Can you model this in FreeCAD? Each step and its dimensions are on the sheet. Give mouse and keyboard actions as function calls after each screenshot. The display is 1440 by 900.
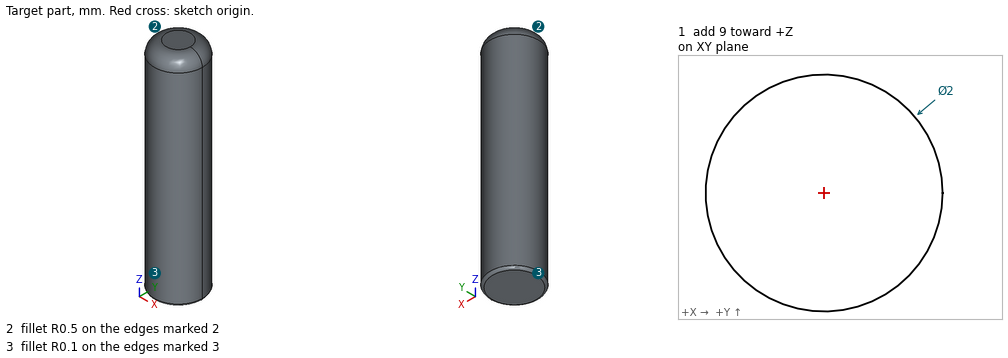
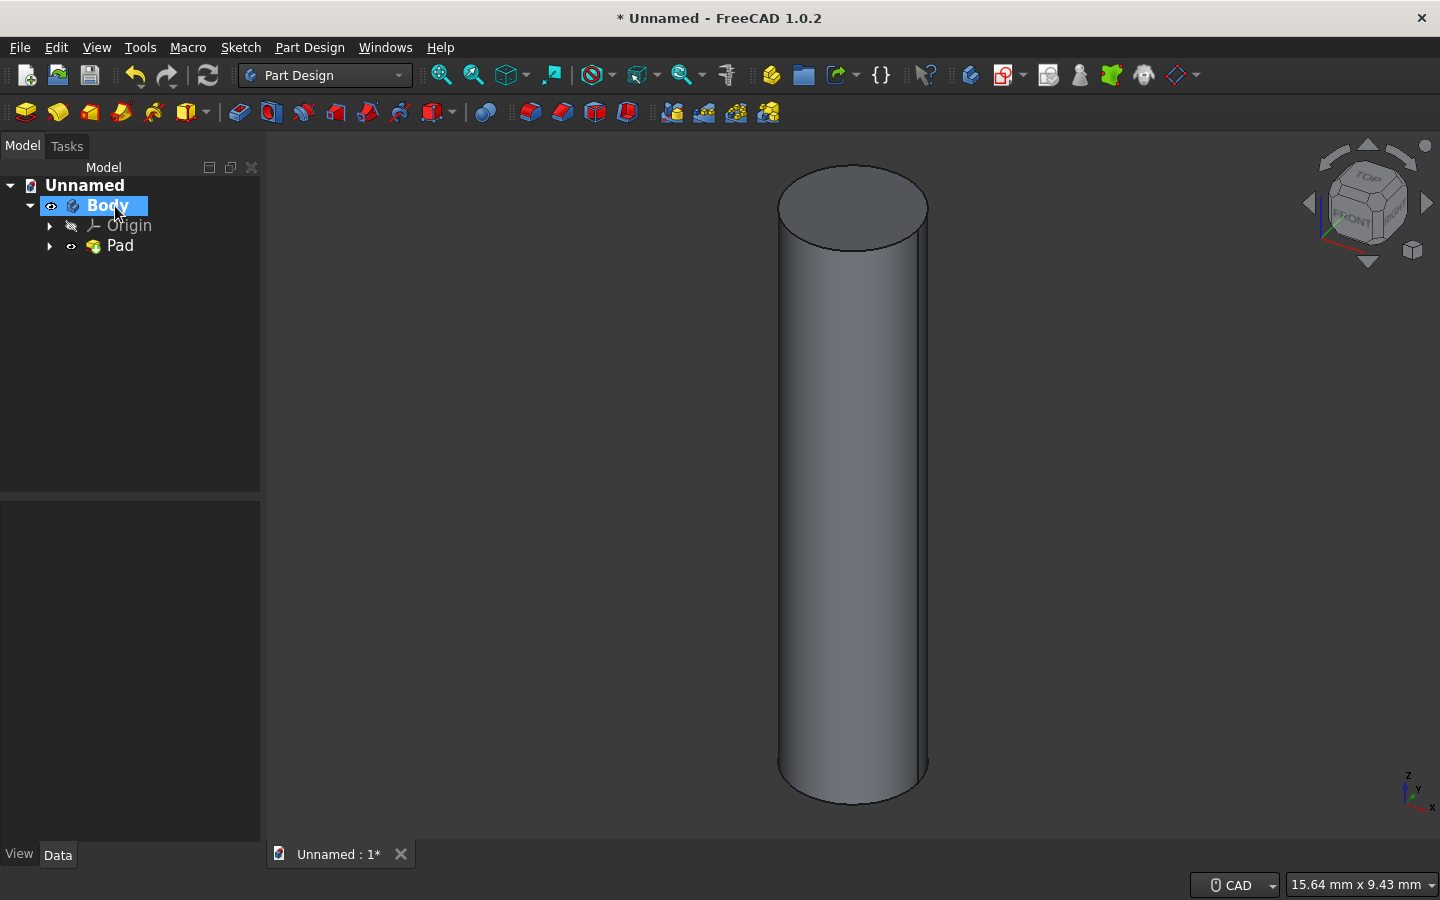
click(778, 212)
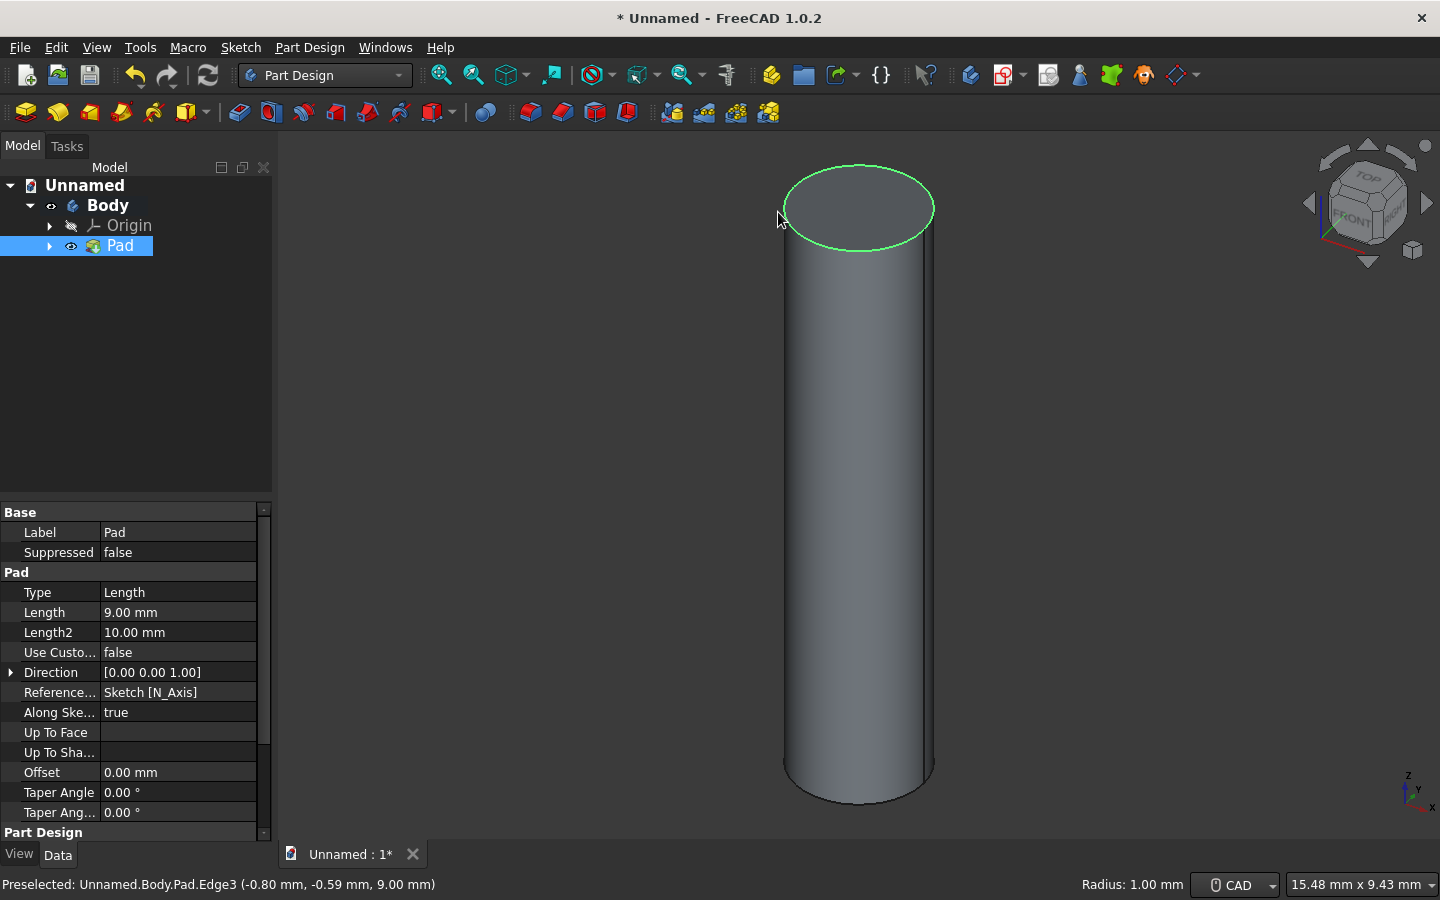
click(532, 112)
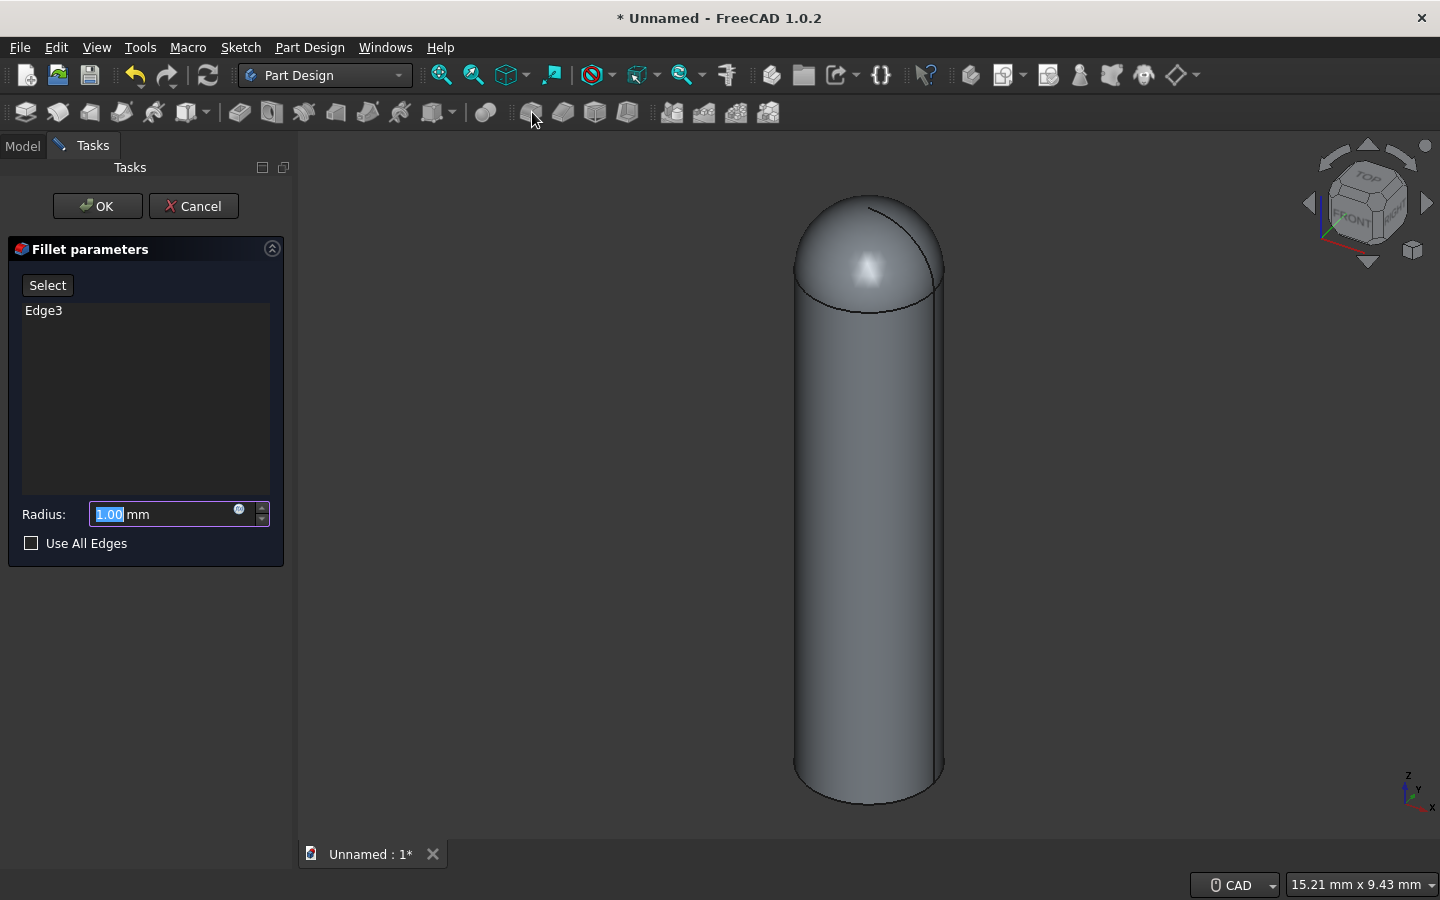
text(0.5)
key(Tab)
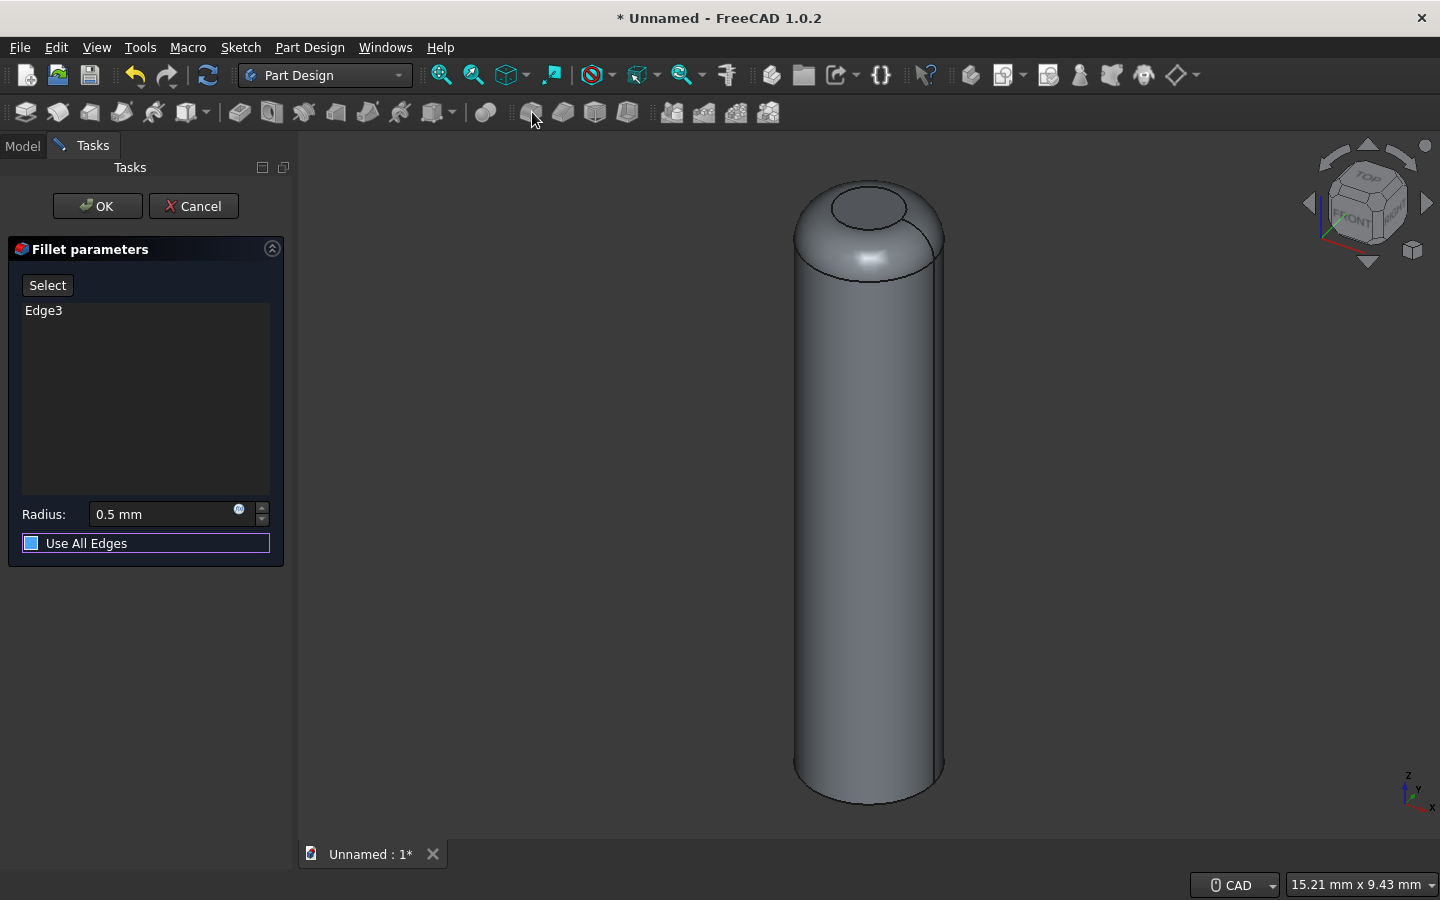
click(98, 206)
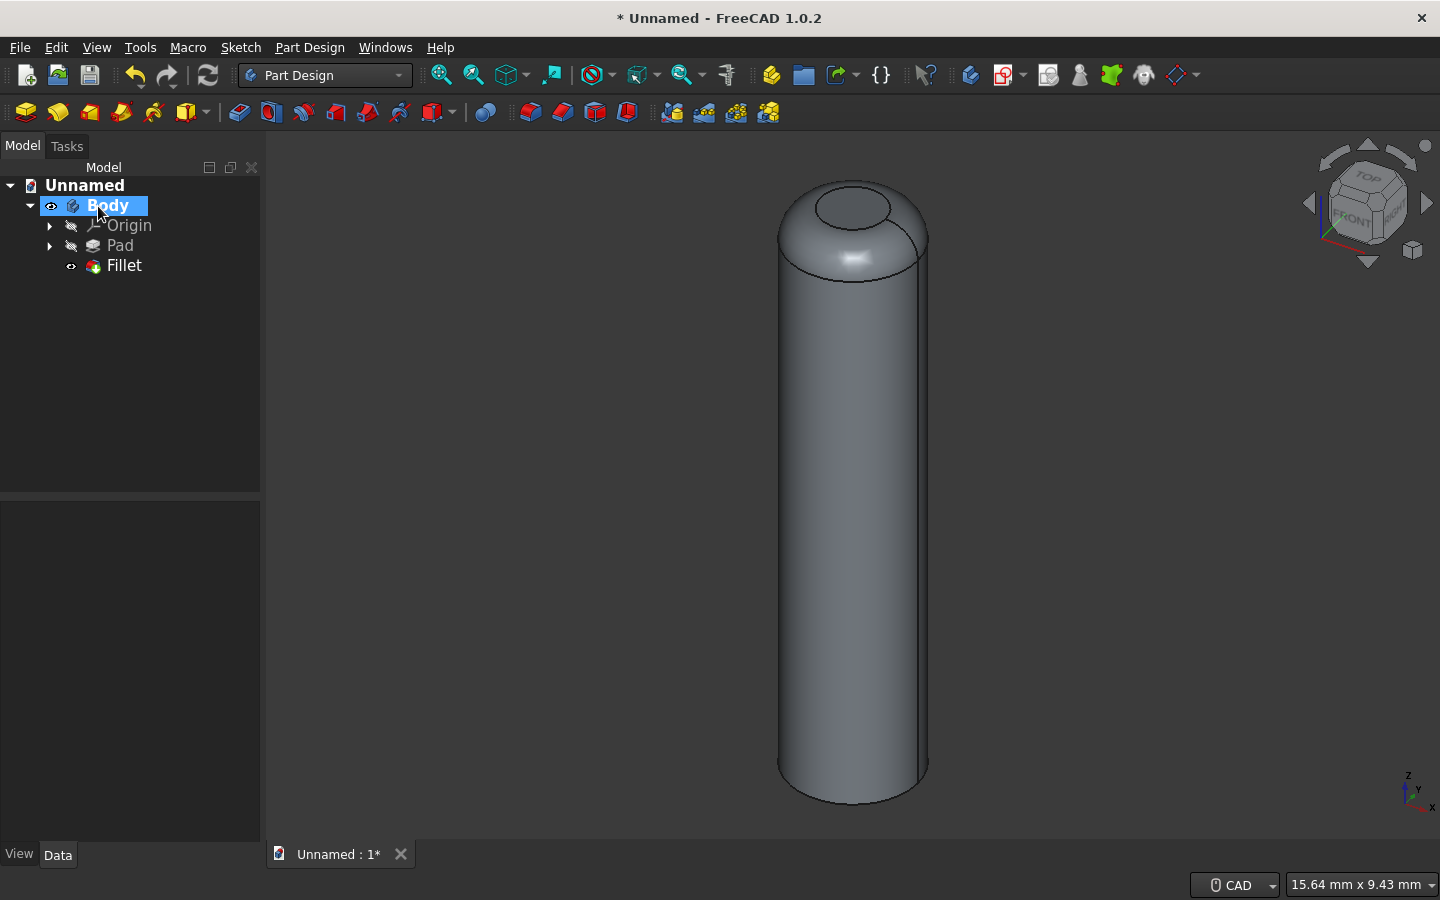
click(797, 790)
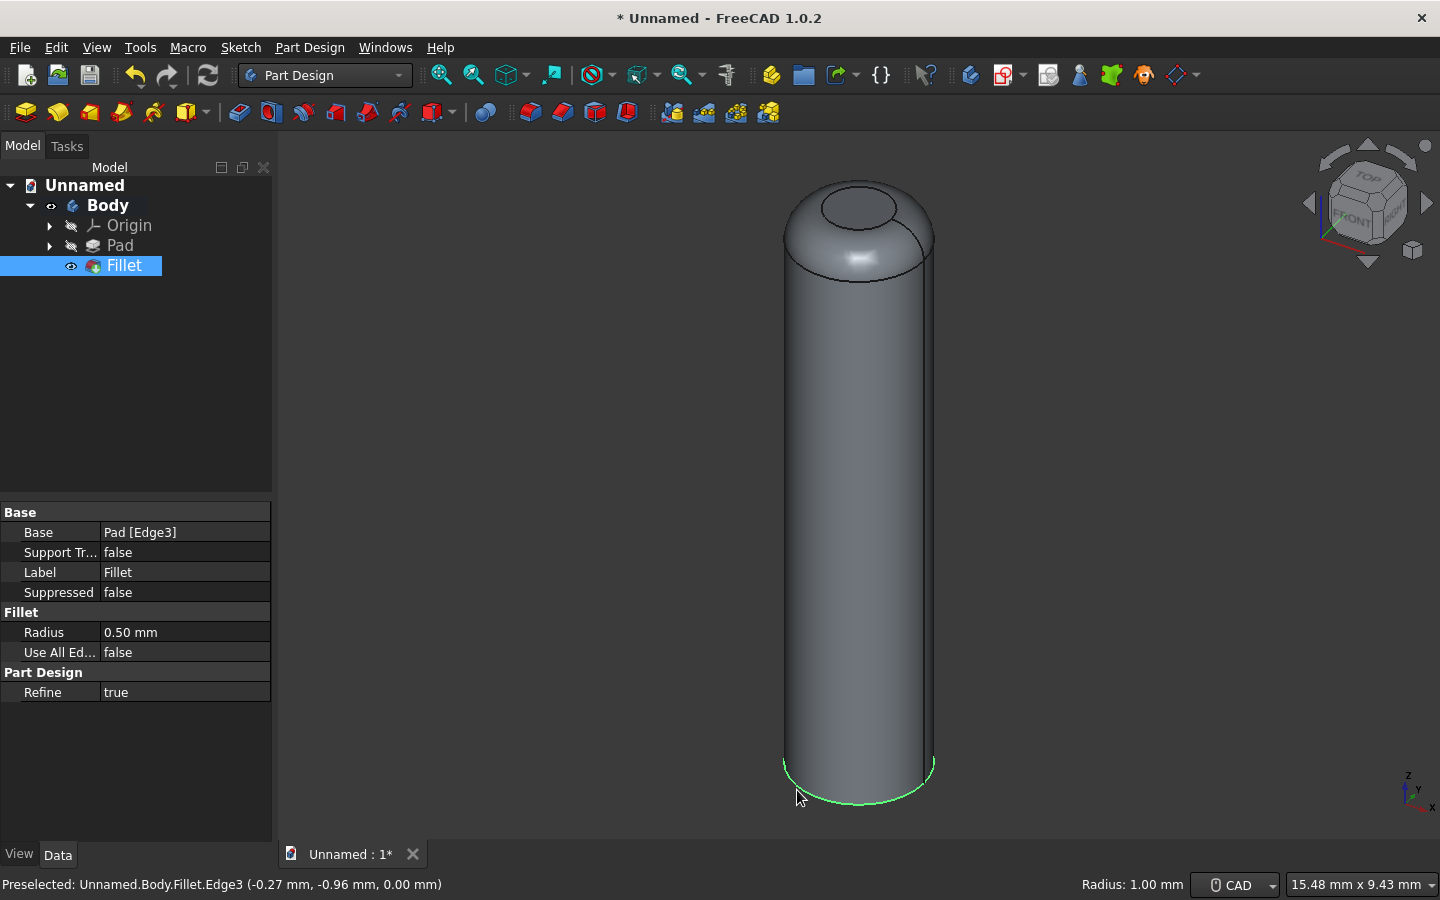
click(532, 112)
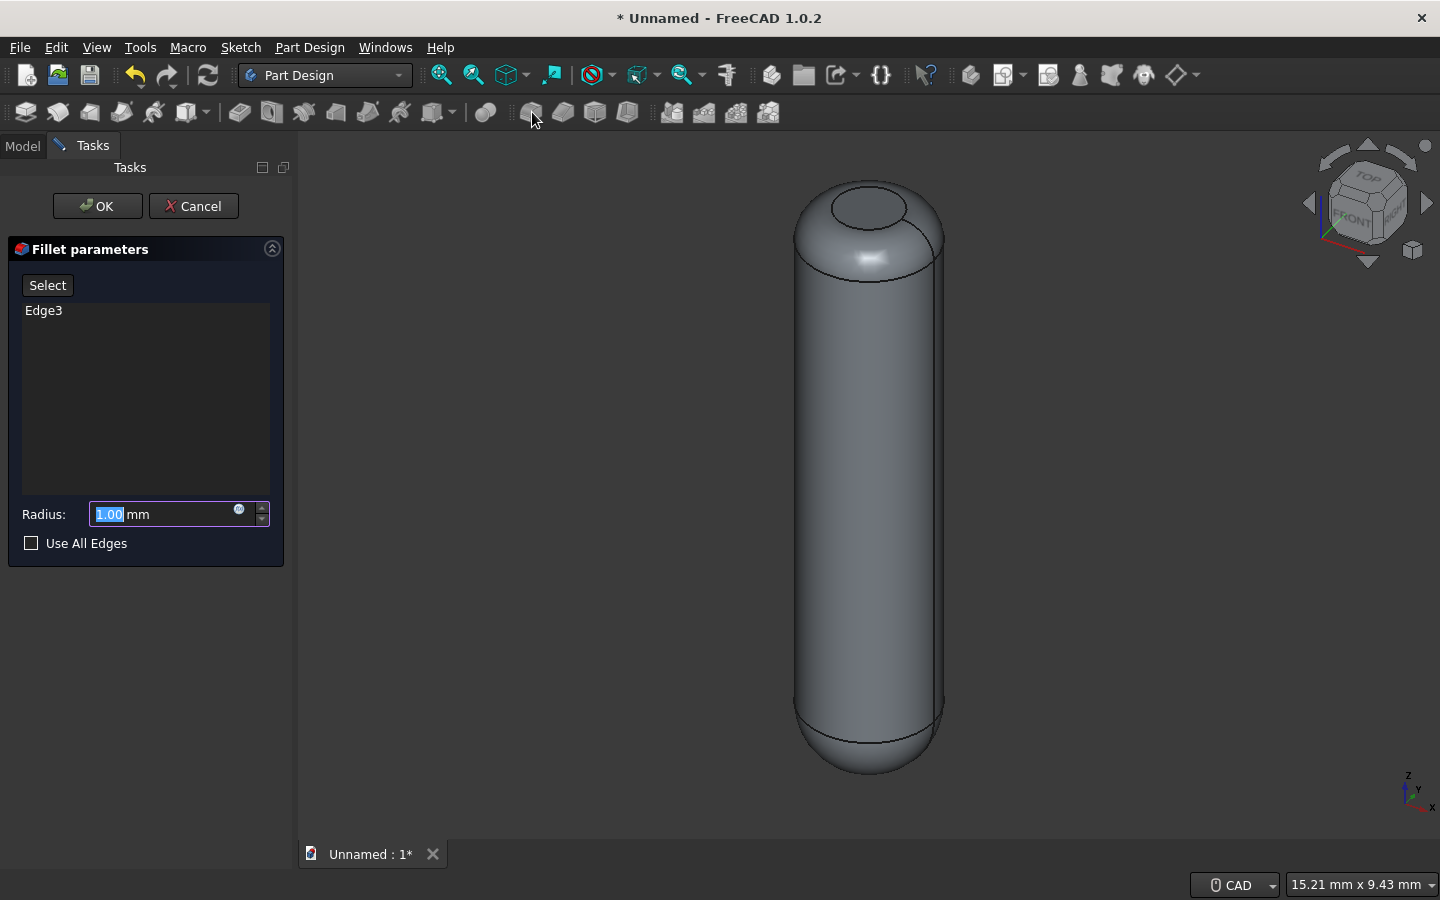
text(0.1)
key(Tab)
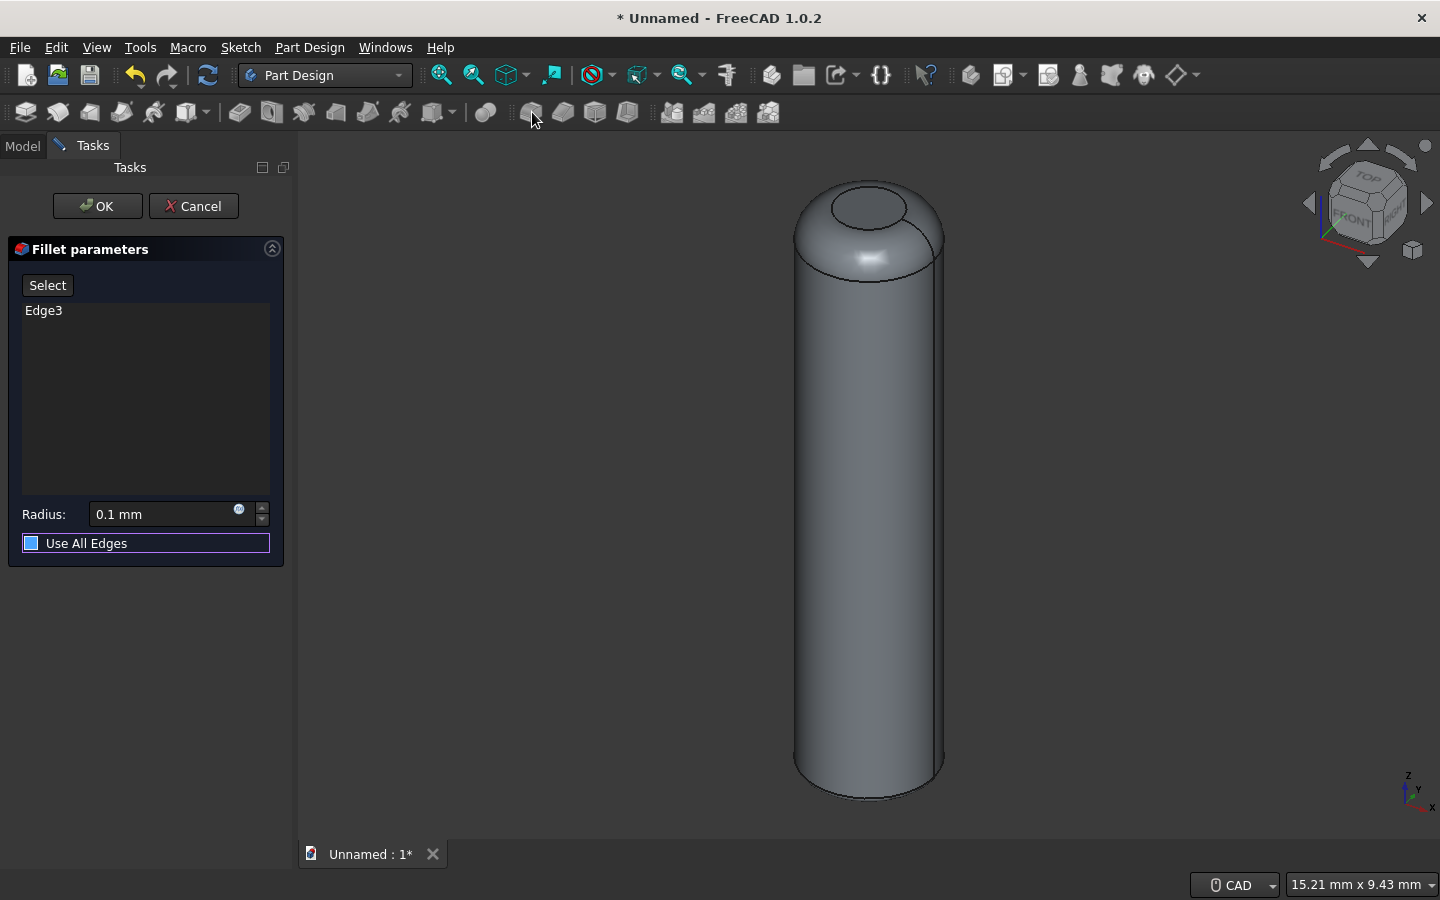
click(98, 206)